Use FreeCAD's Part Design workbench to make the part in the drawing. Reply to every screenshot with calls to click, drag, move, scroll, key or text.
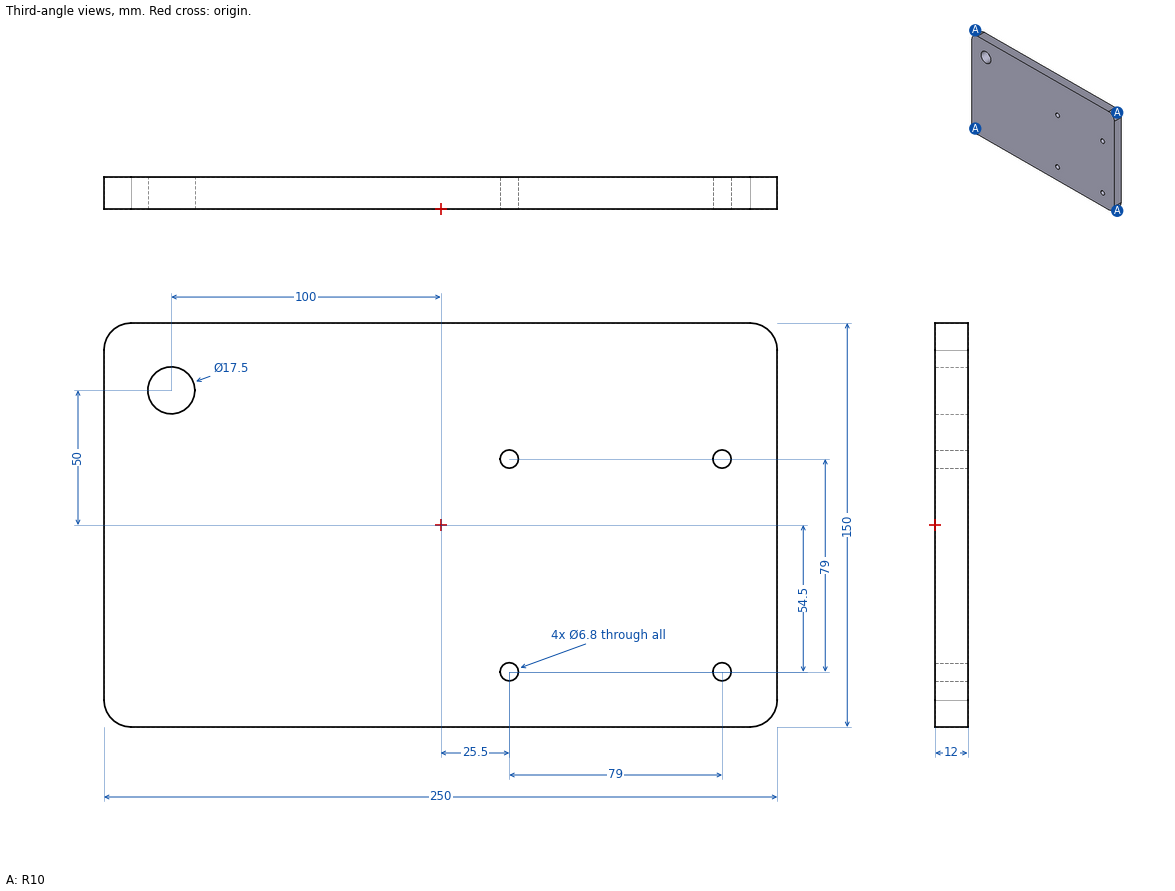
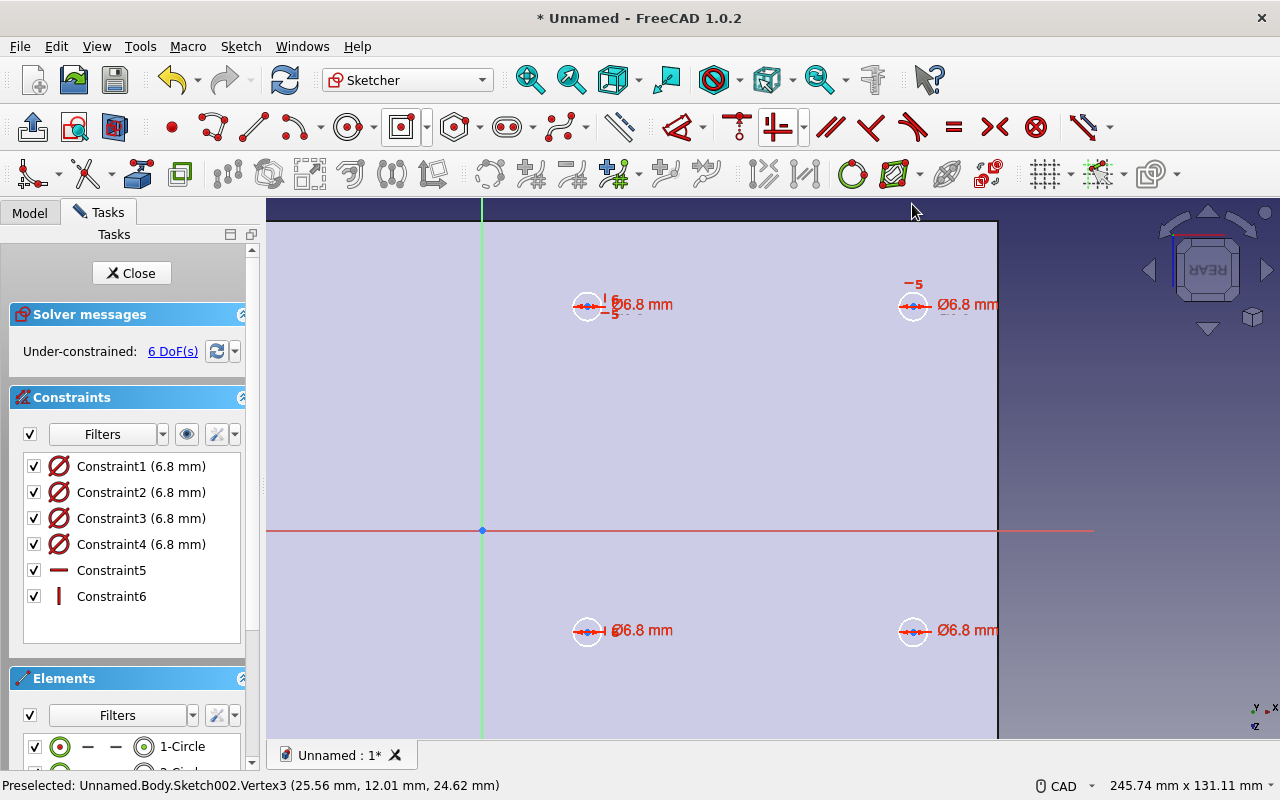
click(913, 307)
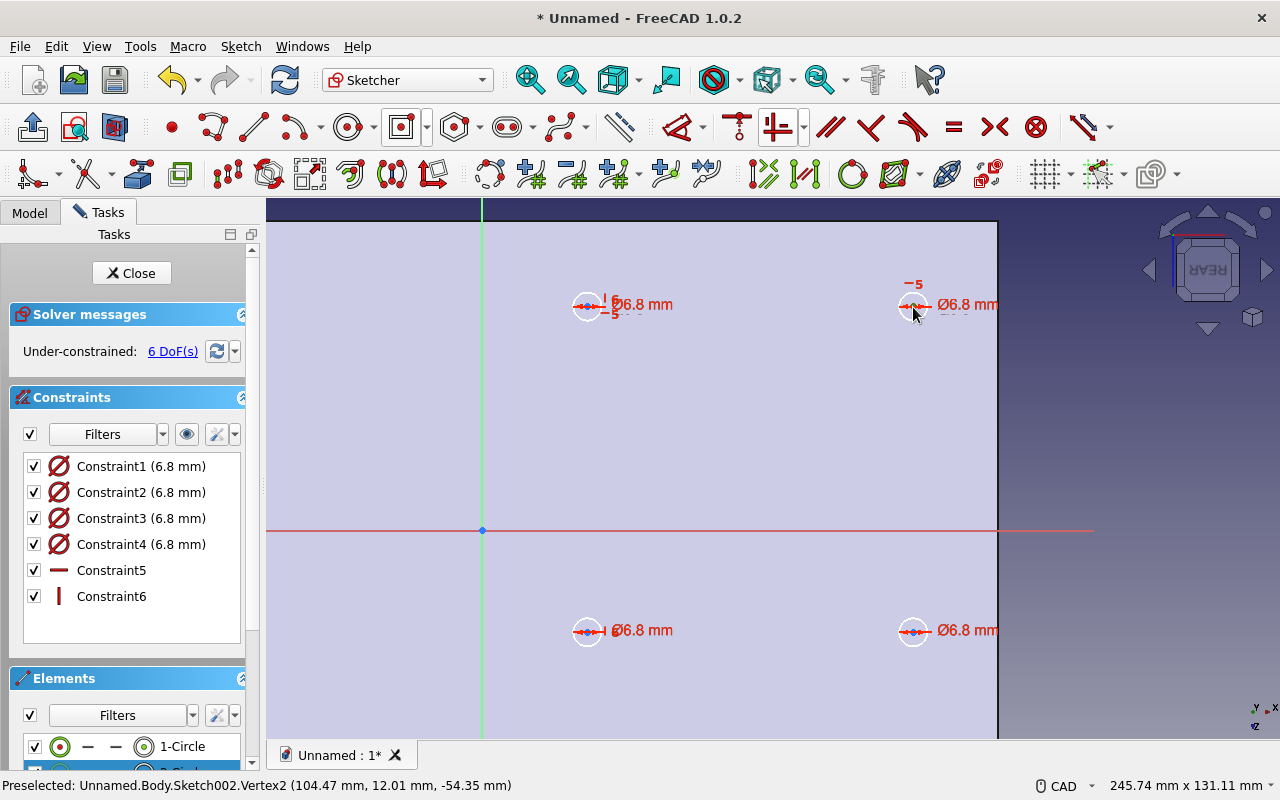
click(913, 632)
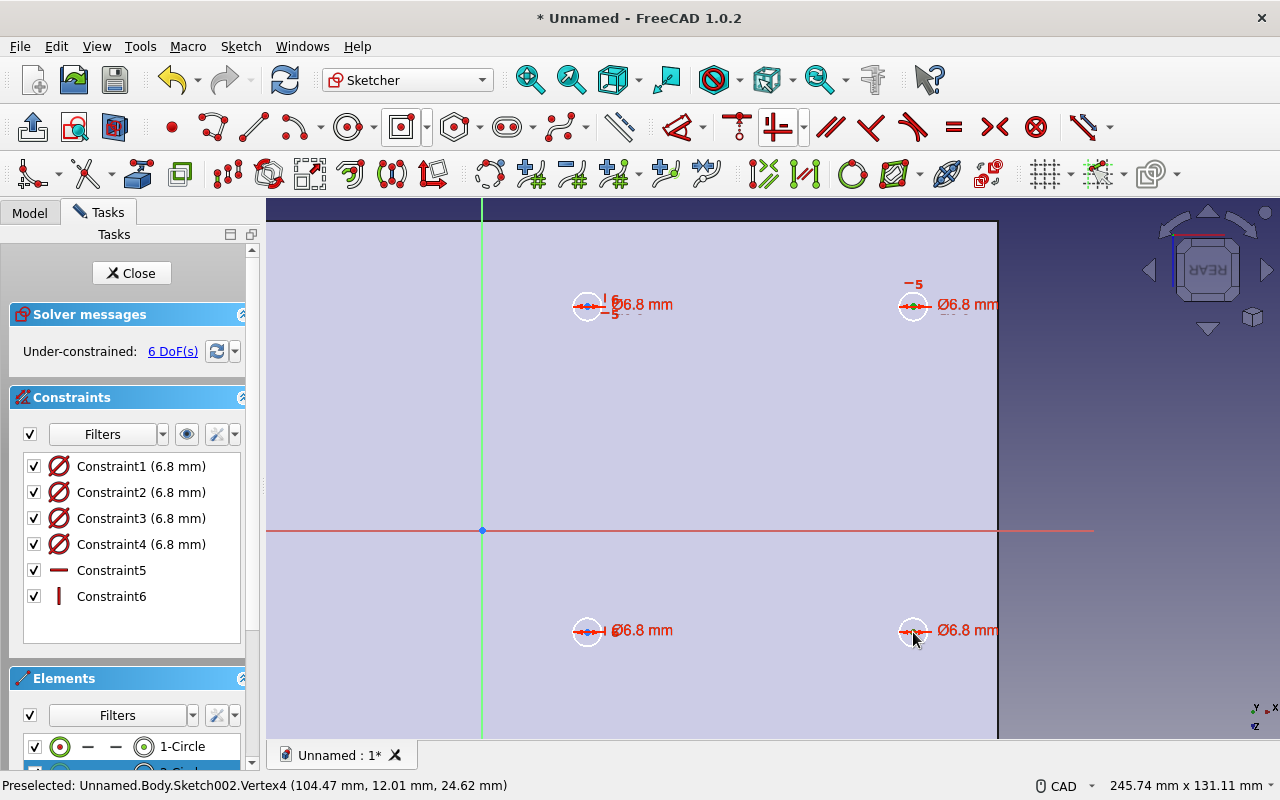
key(v)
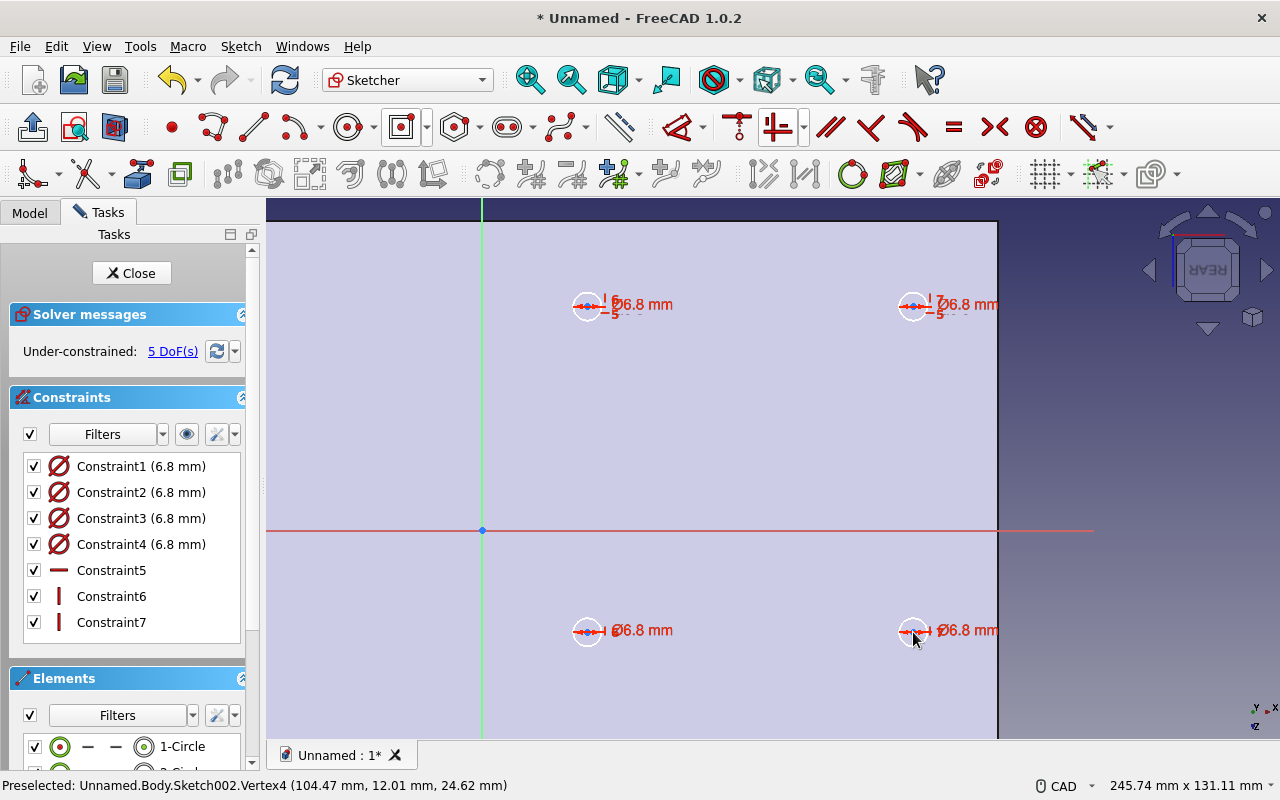
click(587, 632)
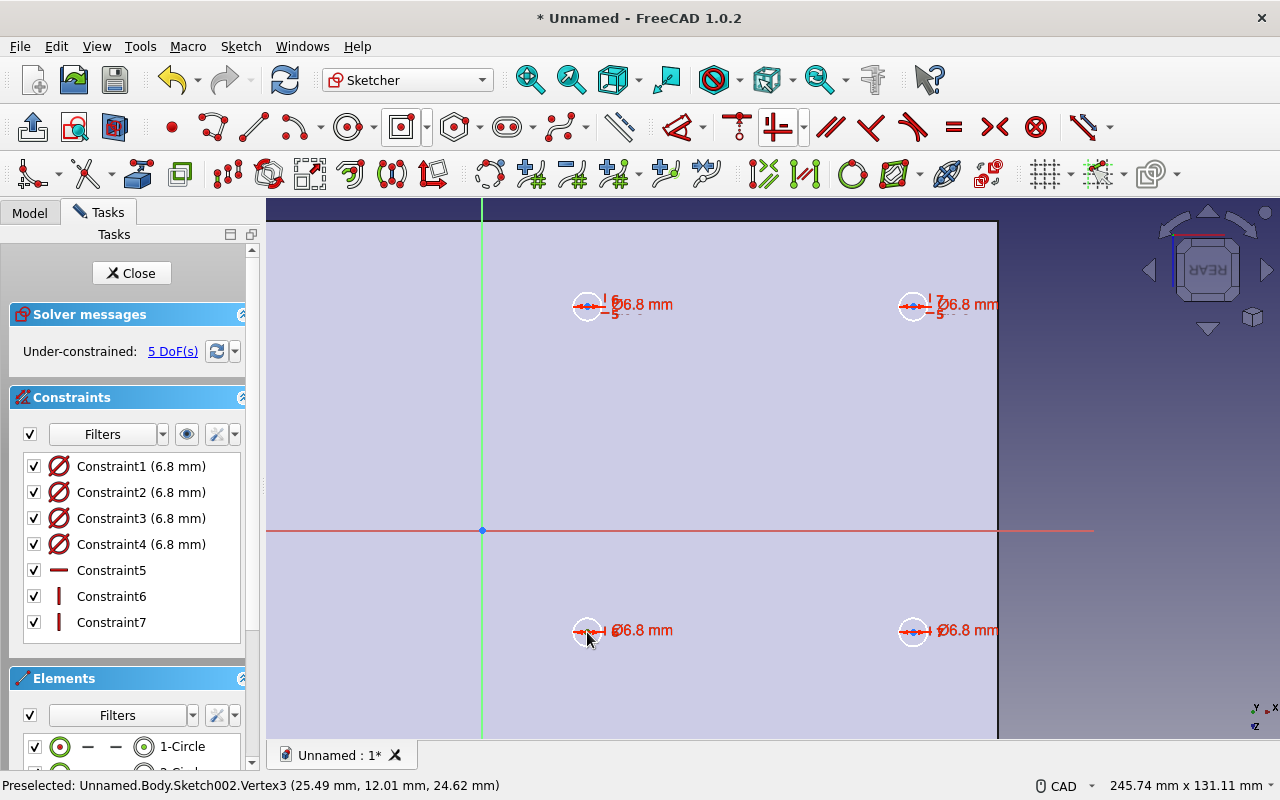
click(913, 632)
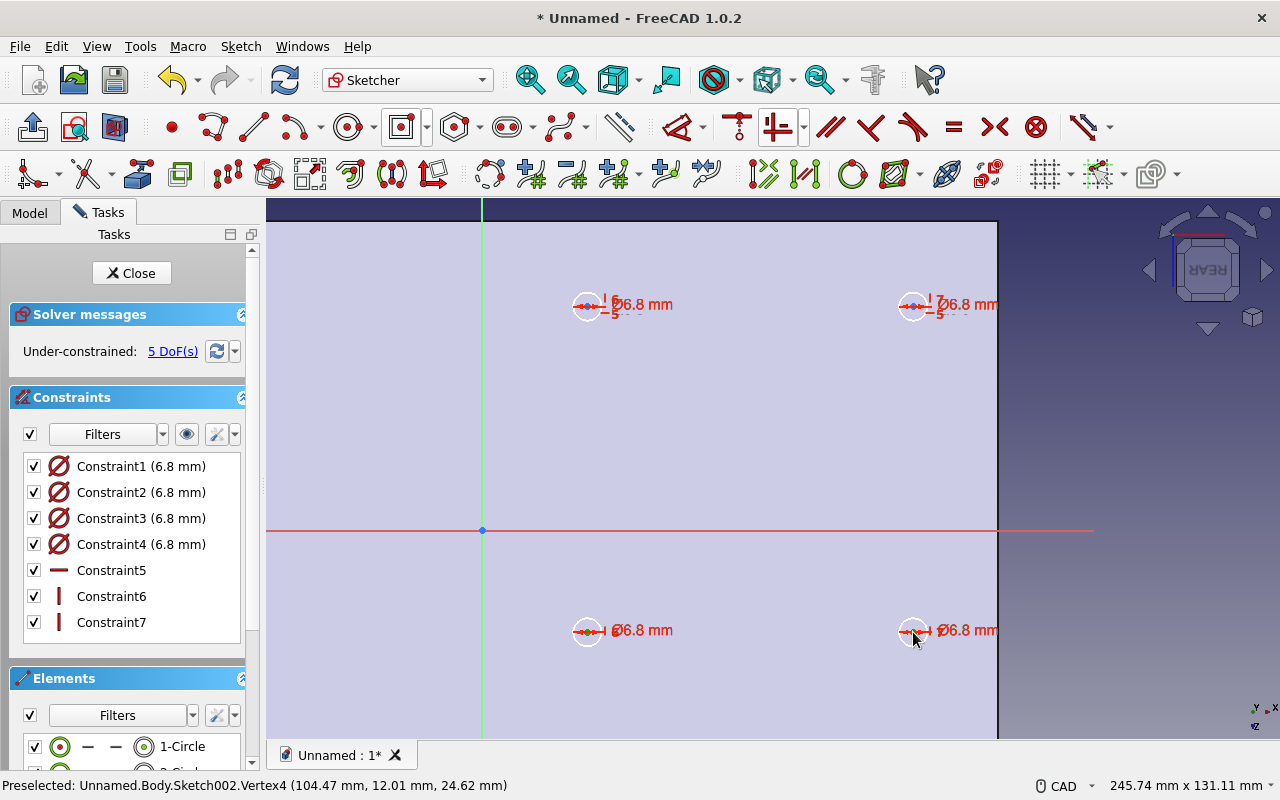
click(804, 128)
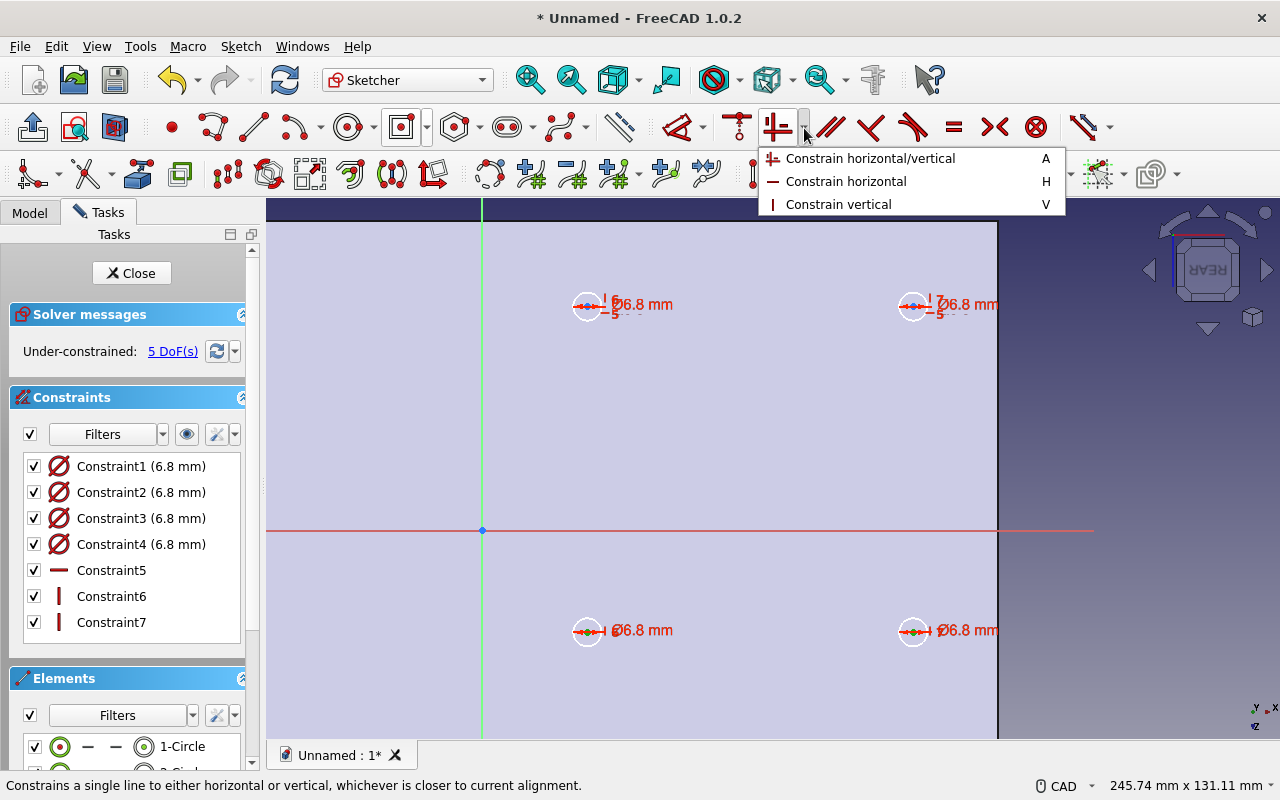
click(912, 182)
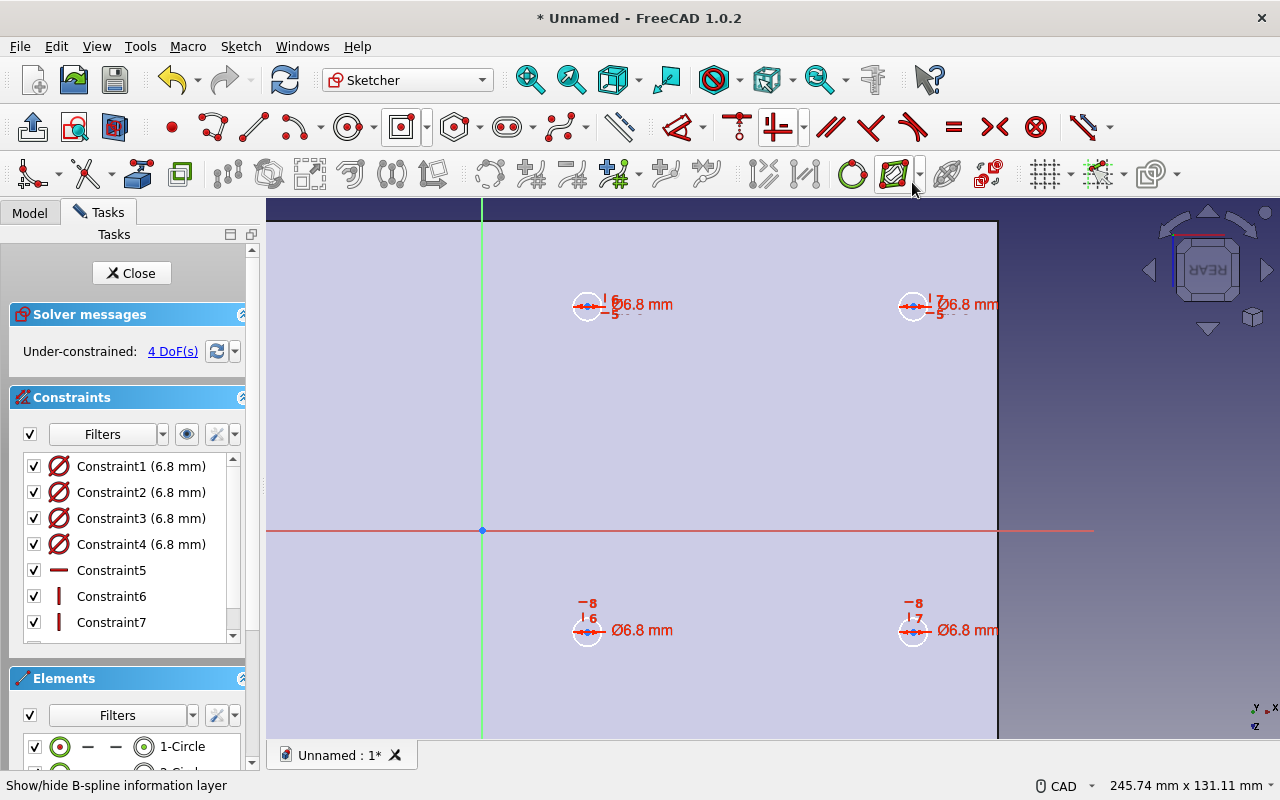
click(676, 128)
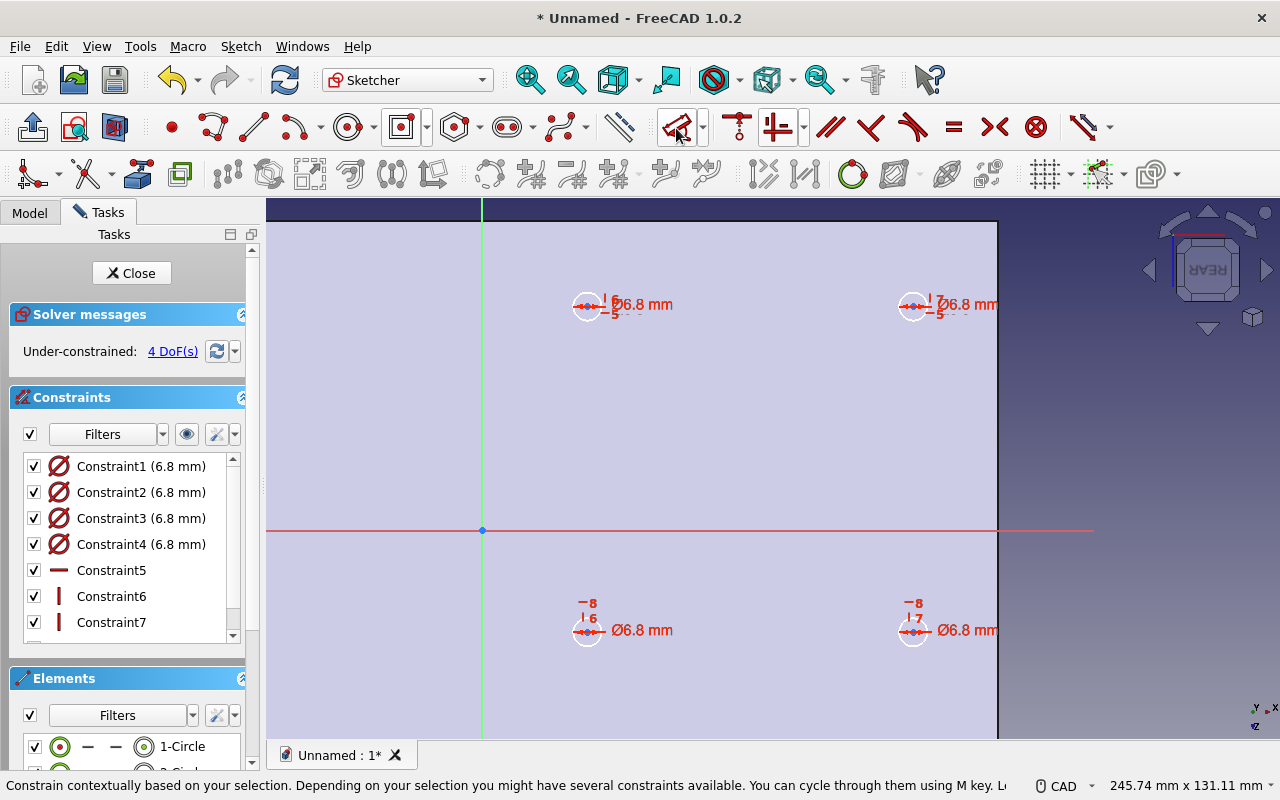
click(587, 307)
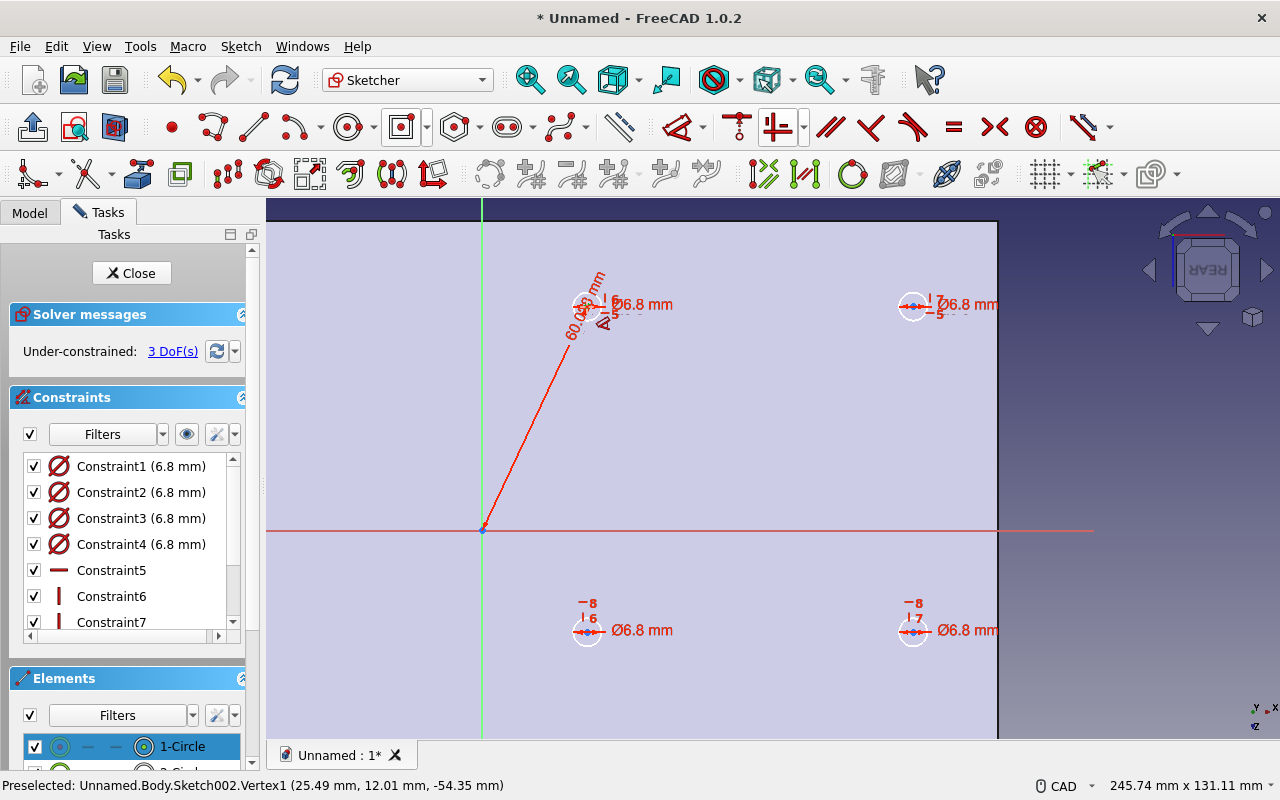
click(913, 307)
click(750, 273)